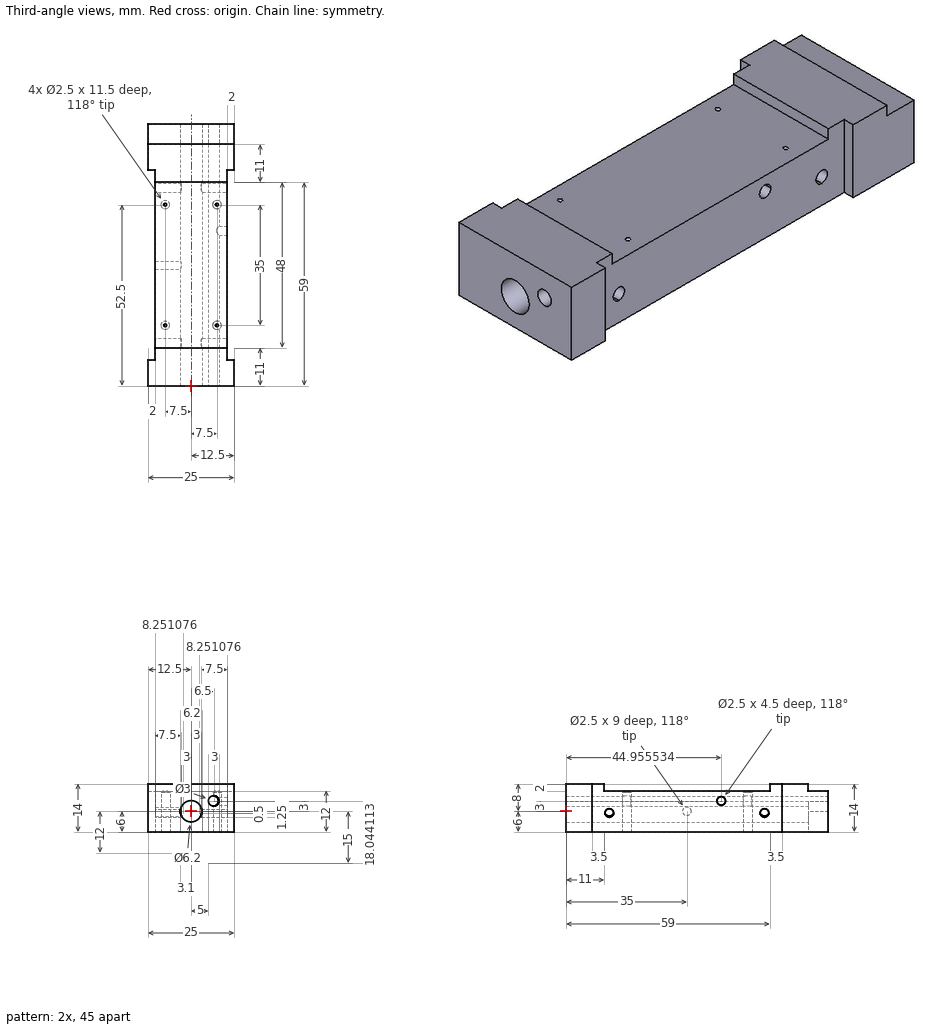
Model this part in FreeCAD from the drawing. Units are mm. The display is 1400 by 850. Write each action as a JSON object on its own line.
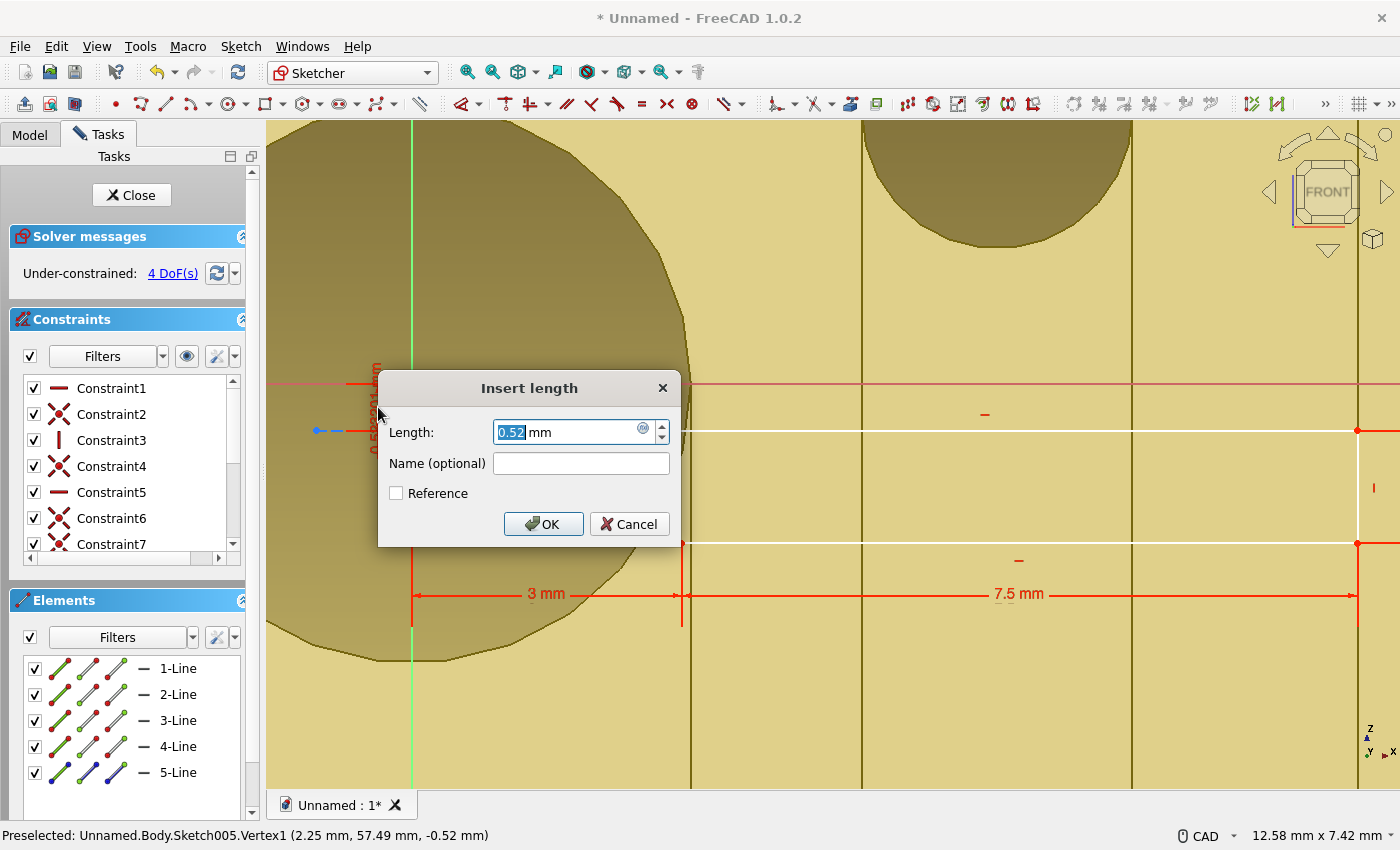
{"action": "type", "text": "0.5"}
{"action": "key", "text": "Return"}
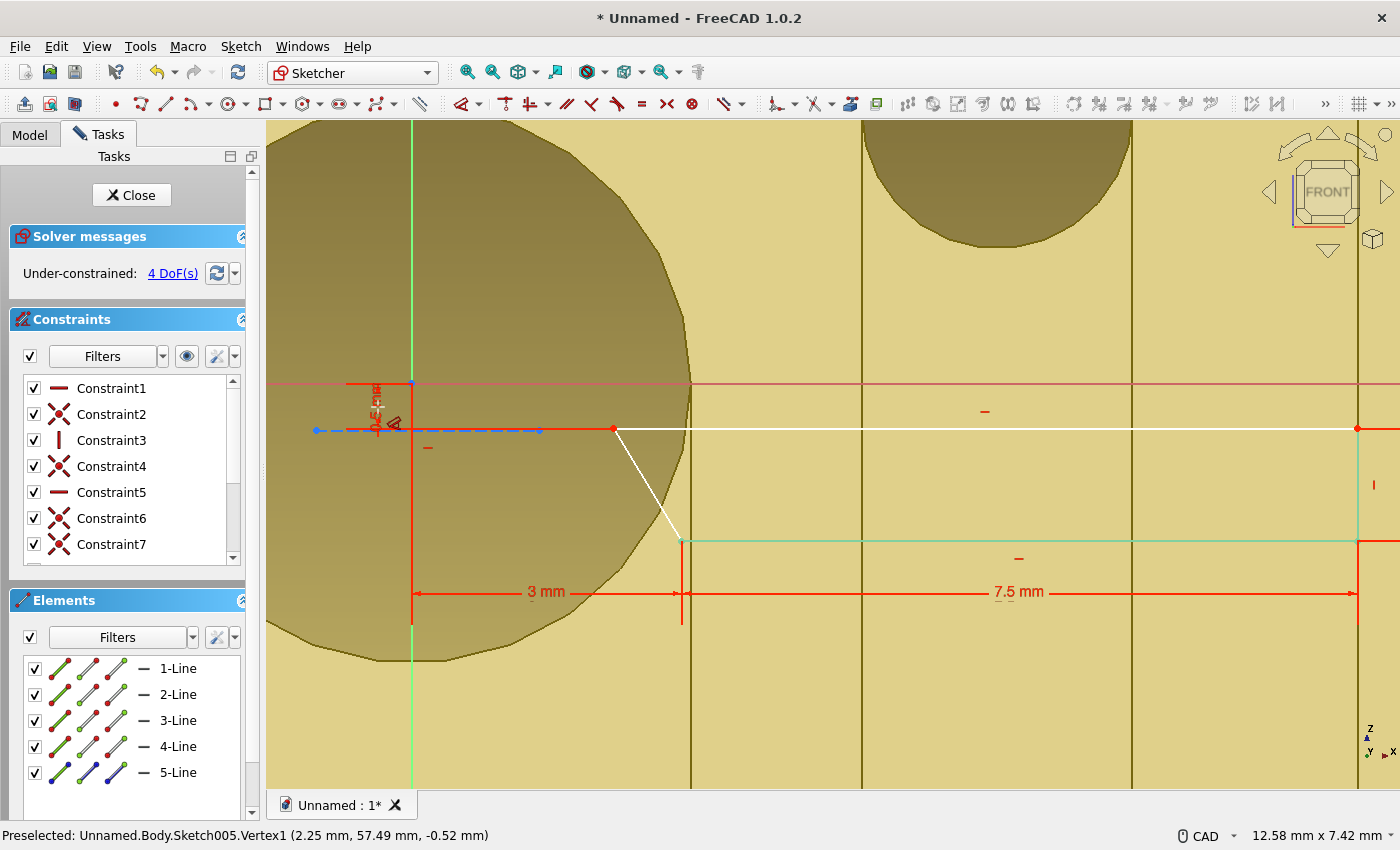
{"action": "left_click", "coordinate": [539, 431]}
{"action": "left_click", "coordinate": [573, 407]}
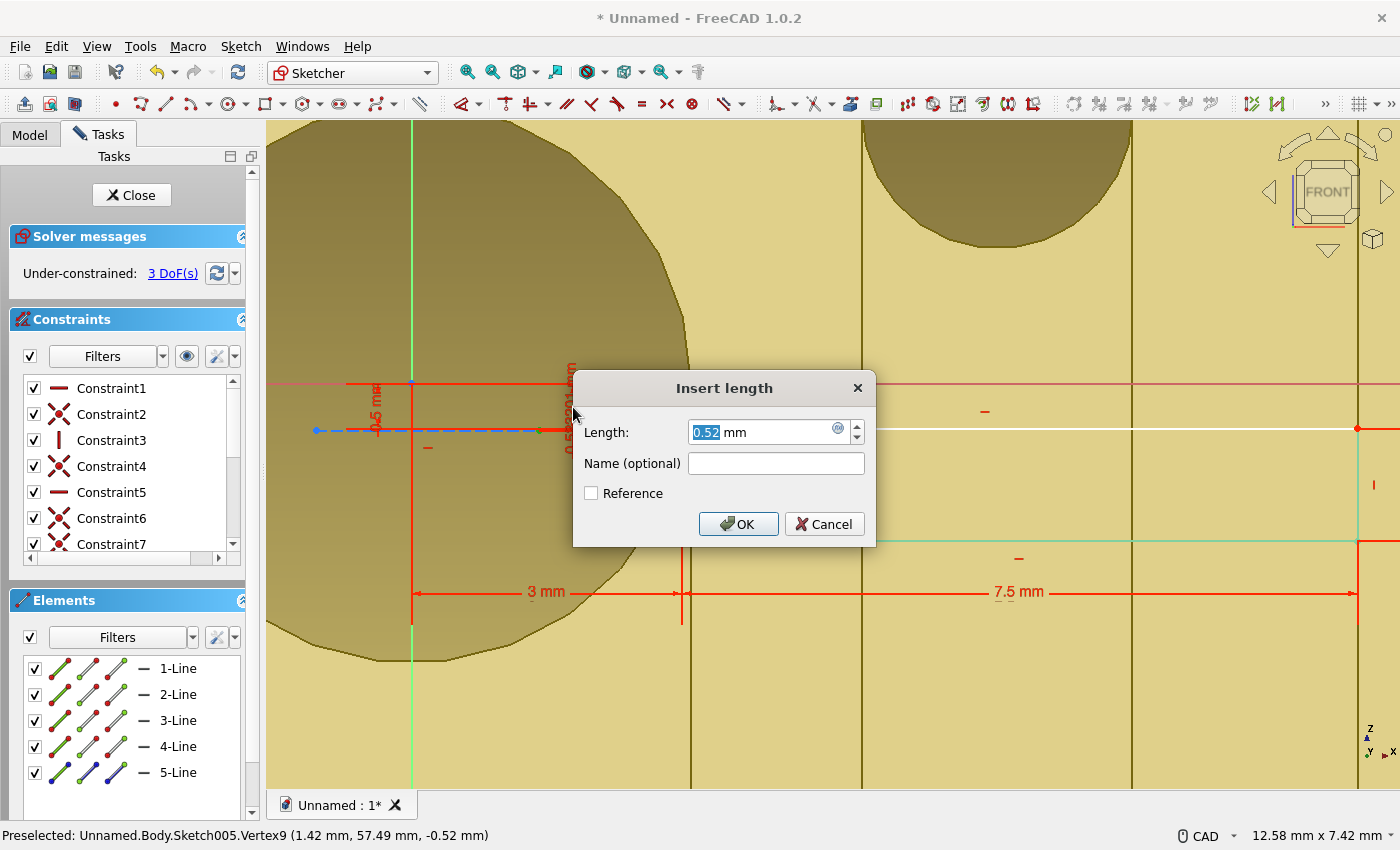
{"action": "type", "text": "0.5"}
{"action": "key", "text": "Return"}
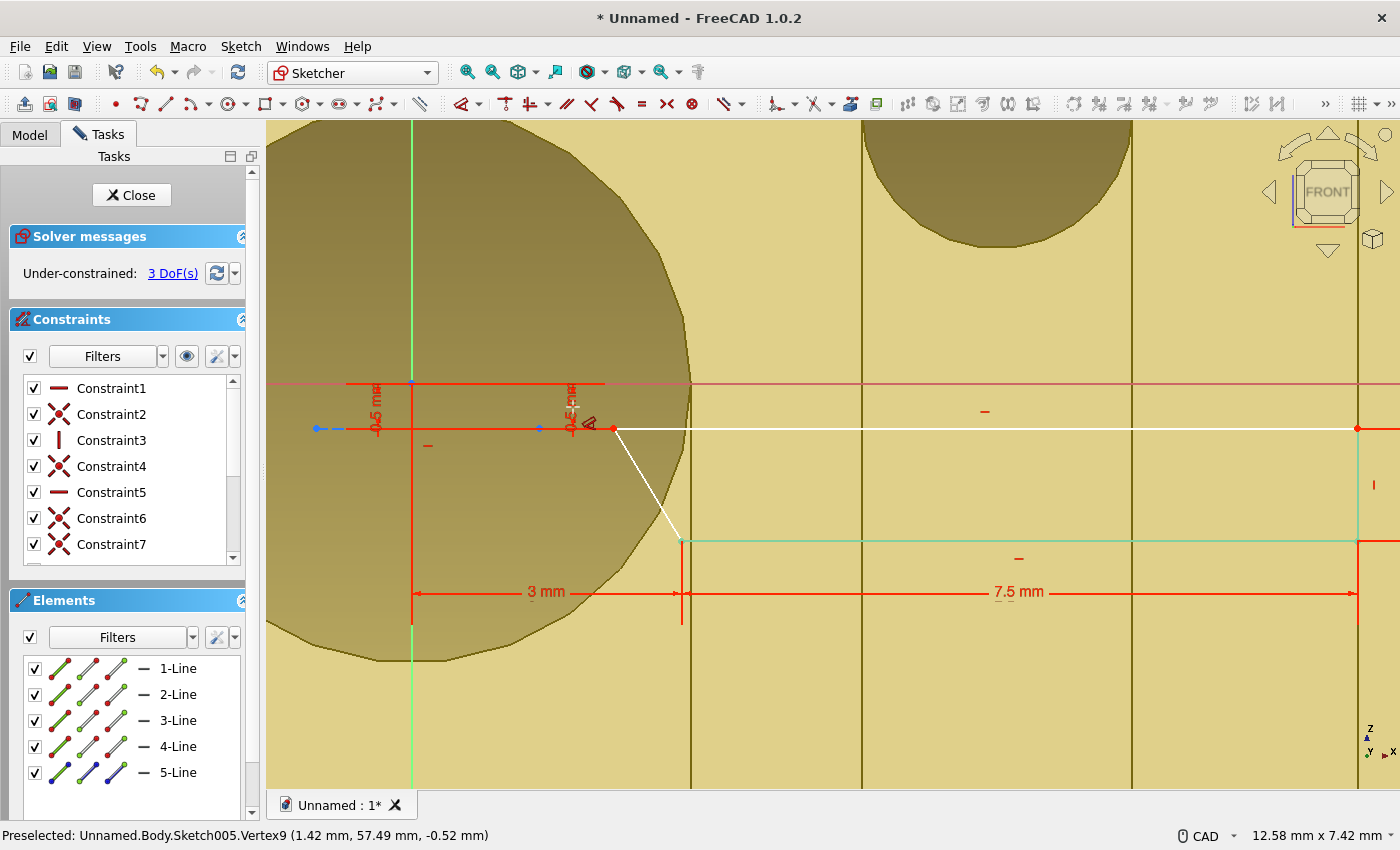
{"action": "left_click", "coordinate": [837, 429]}
{"action": "left_click", "coordinate": [924, 463]}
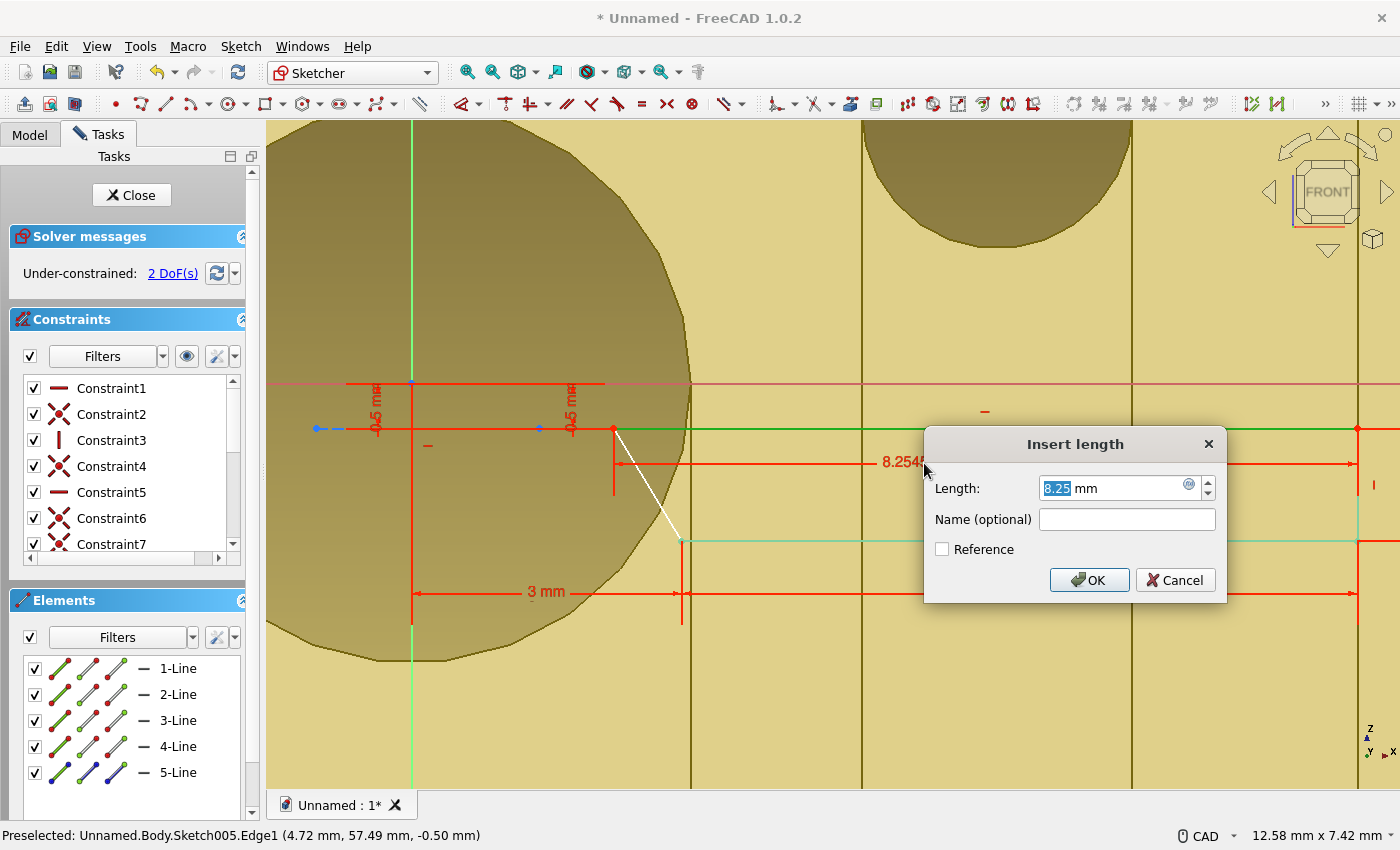
{"action": "type", "text": "8.251076"}
{"action": "key", "text": "Return"}
{"action": "key", "text": "Escape"}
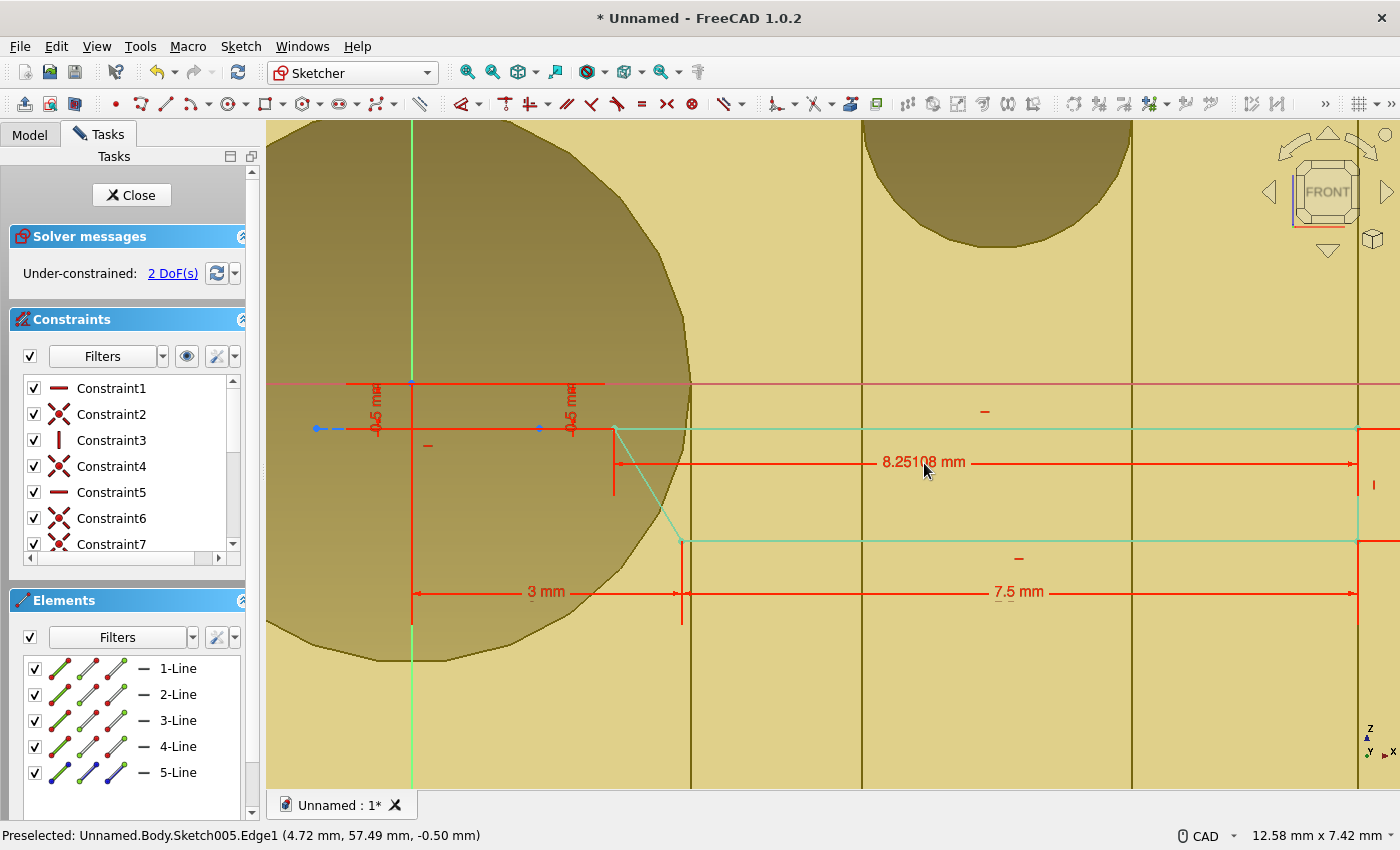
{"action": "left_click", "coordinate": [132, 195]}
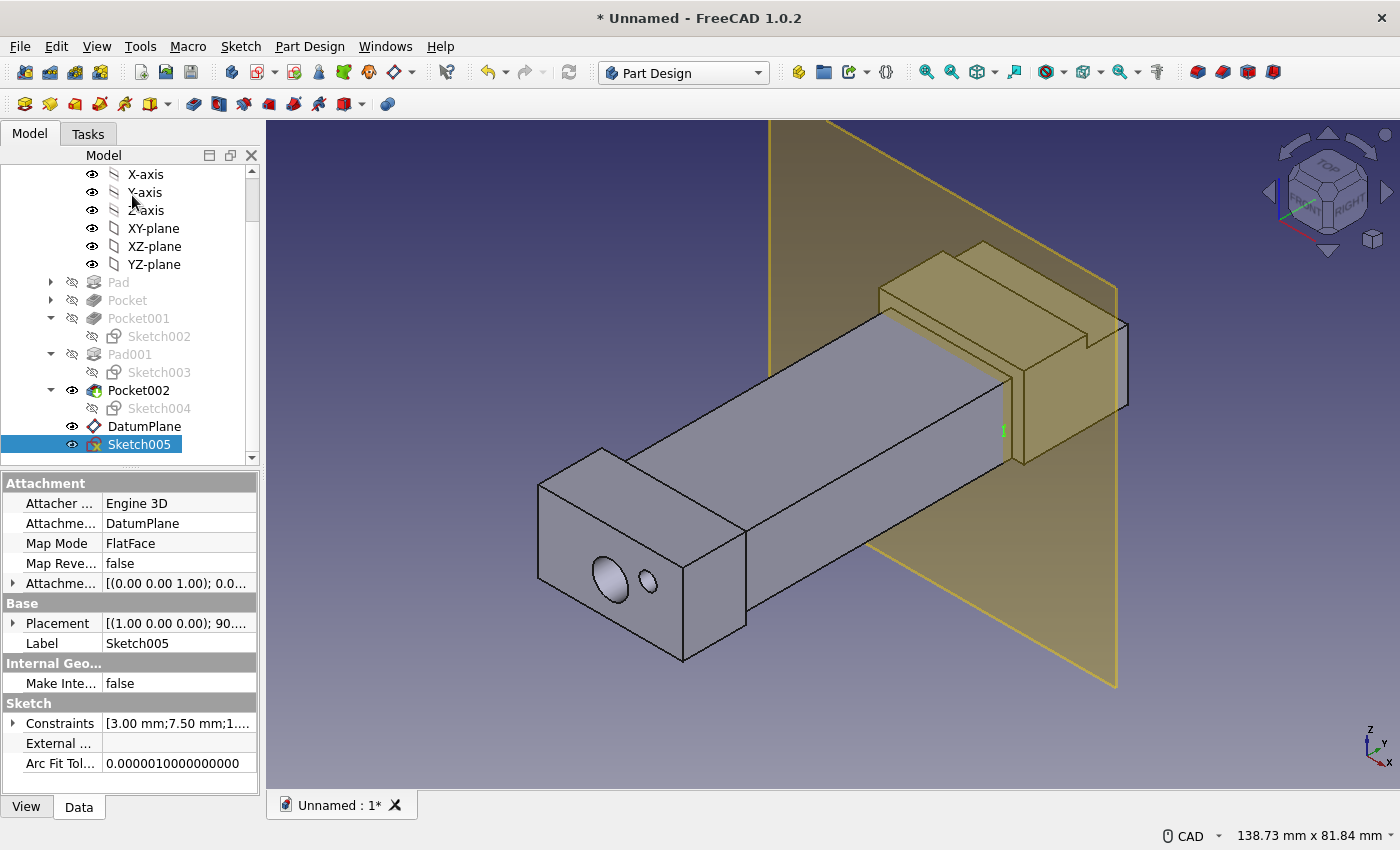
{"action": "left_click", "coordinate": [244, 104]}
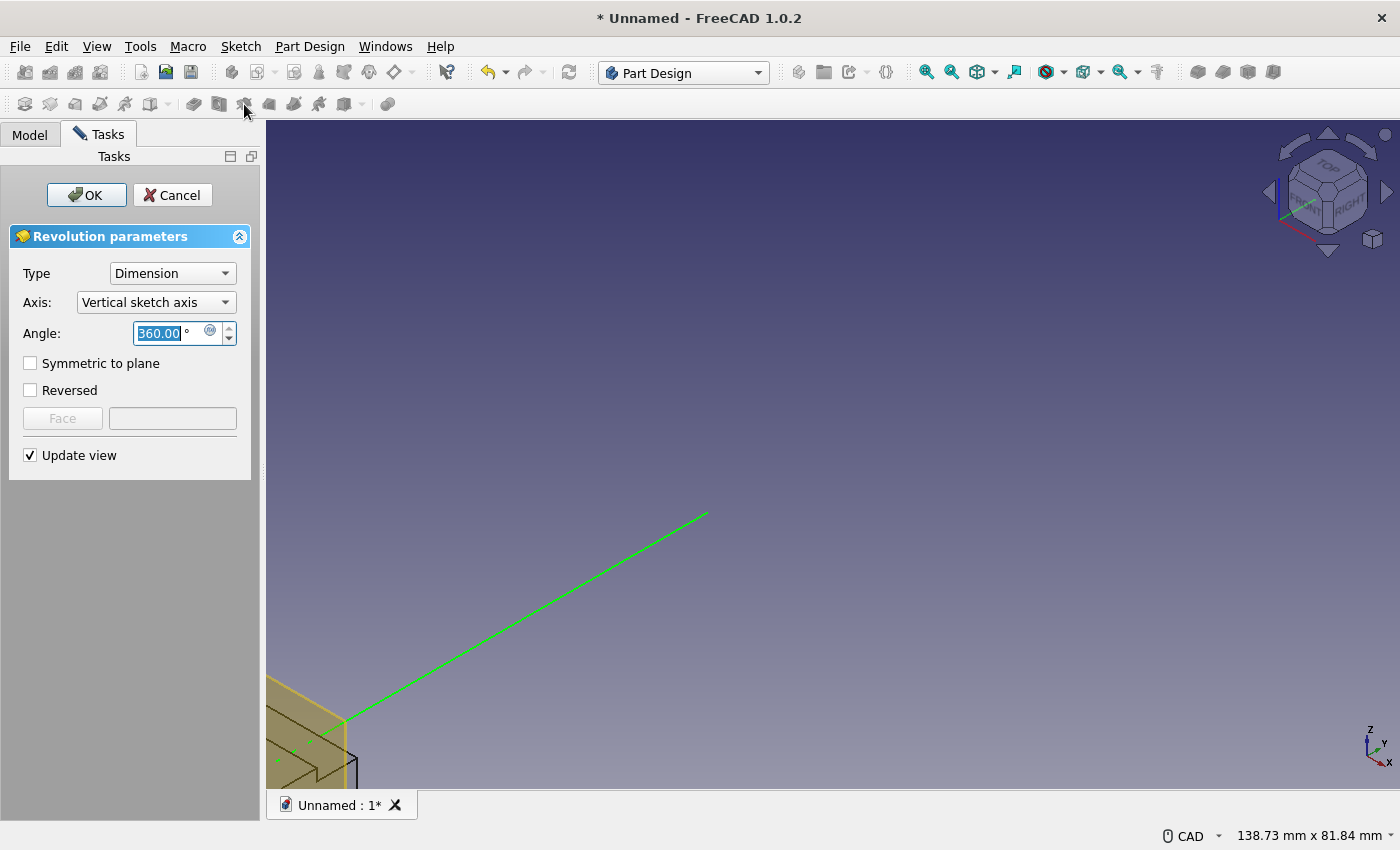
{"action": "left_click", "coordinate": [157, 302]}